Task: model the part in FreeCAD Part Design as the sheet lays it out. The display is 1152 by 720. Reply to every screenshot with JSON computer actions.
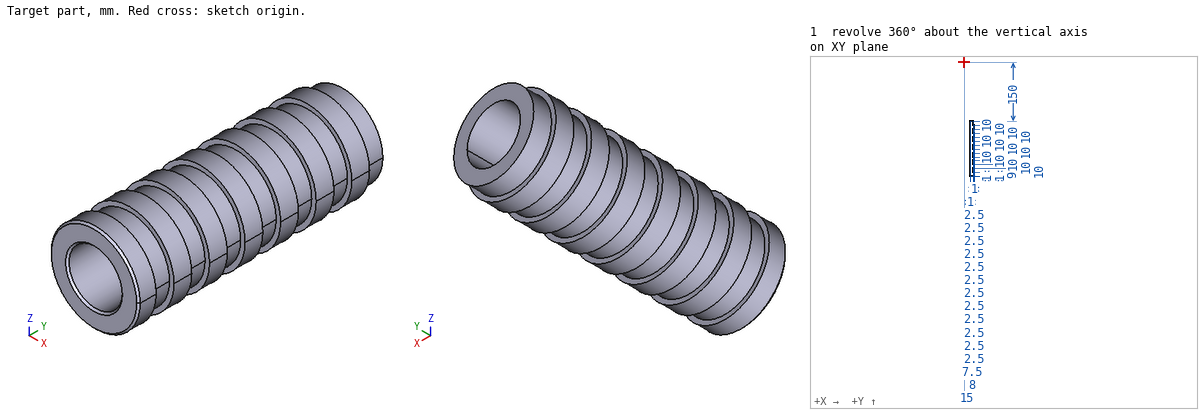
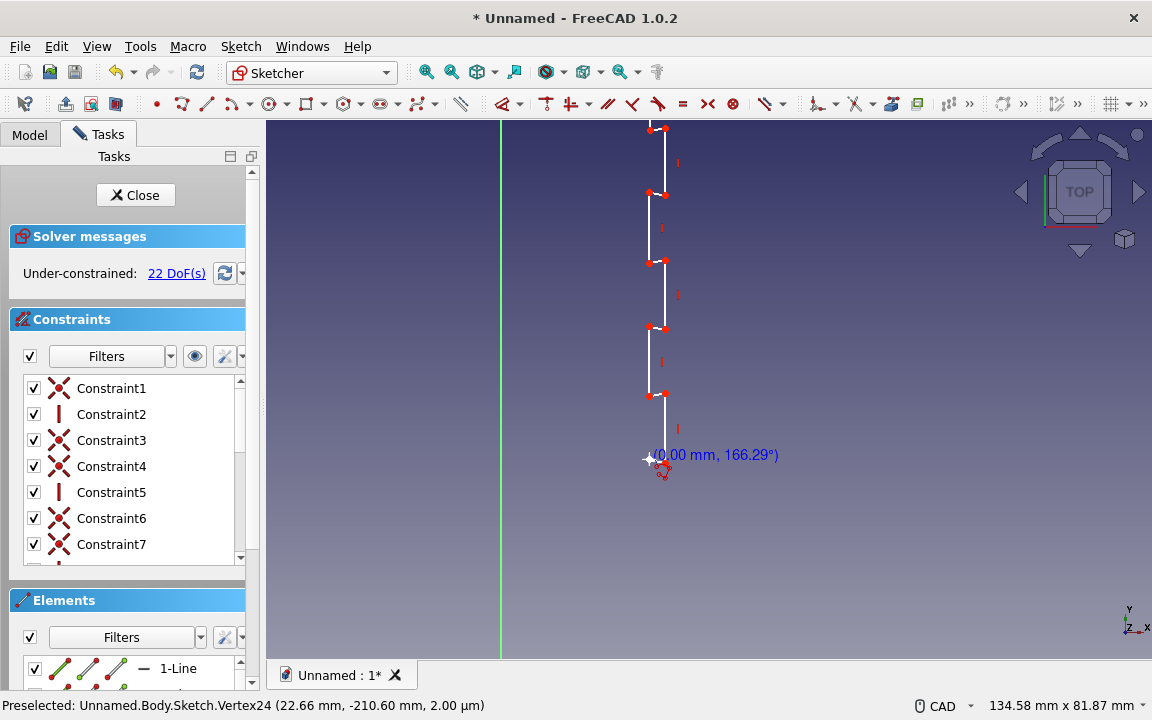
{"action": "scroll", "coordinate": [652, 461], "scroll_direction": "down", "scroll_amount": 9}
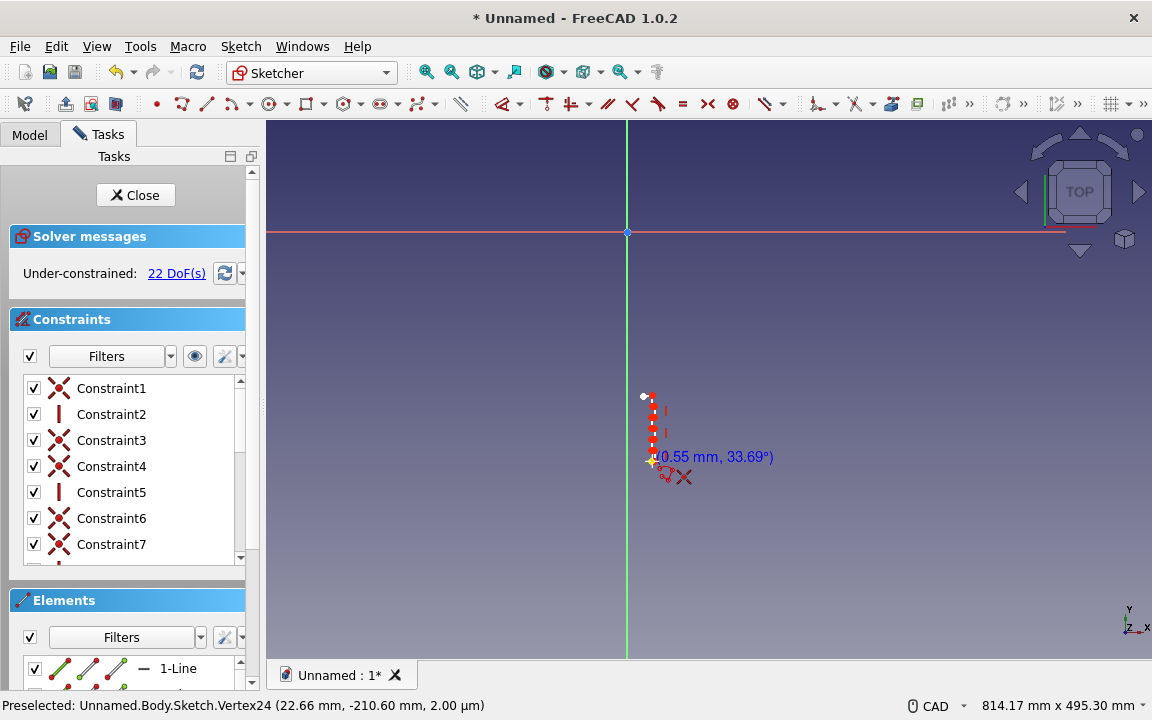
{"action": "scroll", "coordinate": [652, 472], "scroll_direction": "up", "scroll_amount": 2}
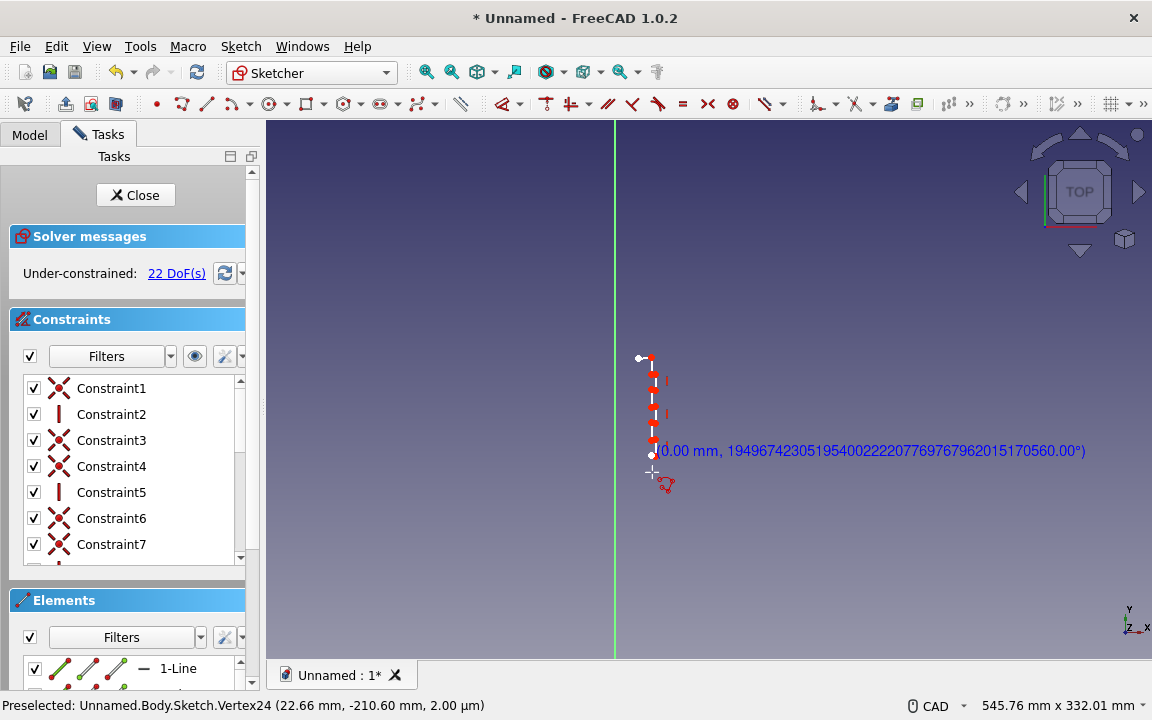
{"action": "left_click", "coordinate": [652, 471]}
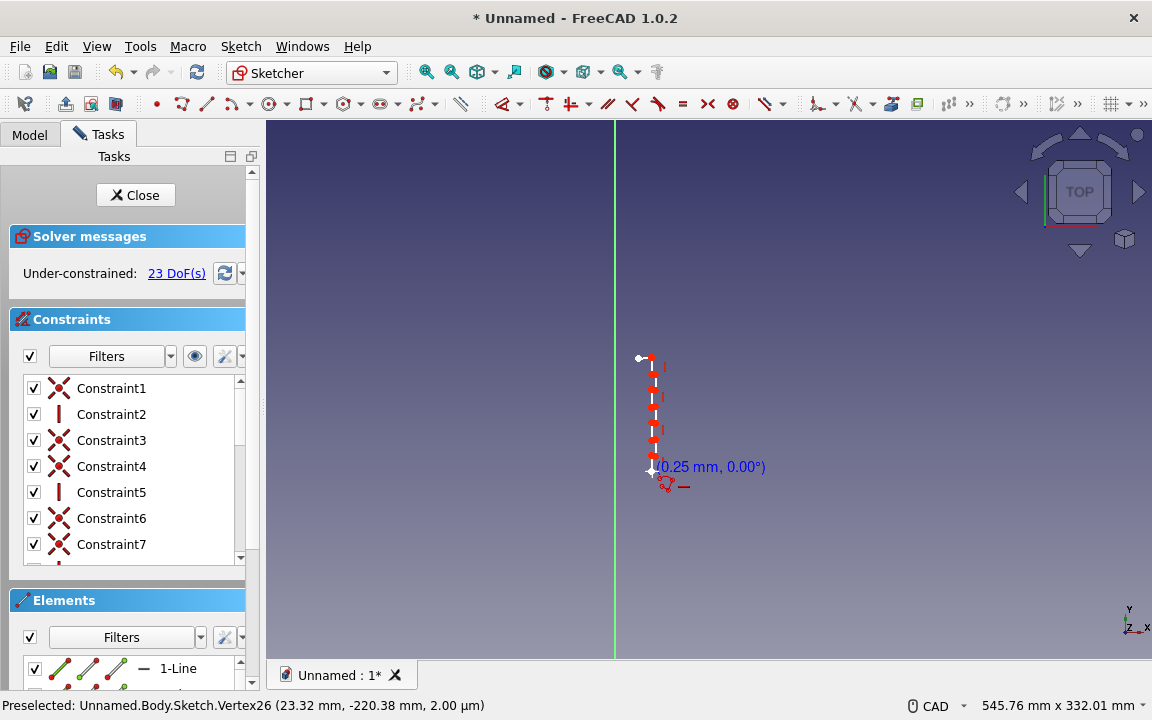
{"action": "scroll", "coordinate": [656, 471], "scroll_direction": "up", "scroll_amount": 7}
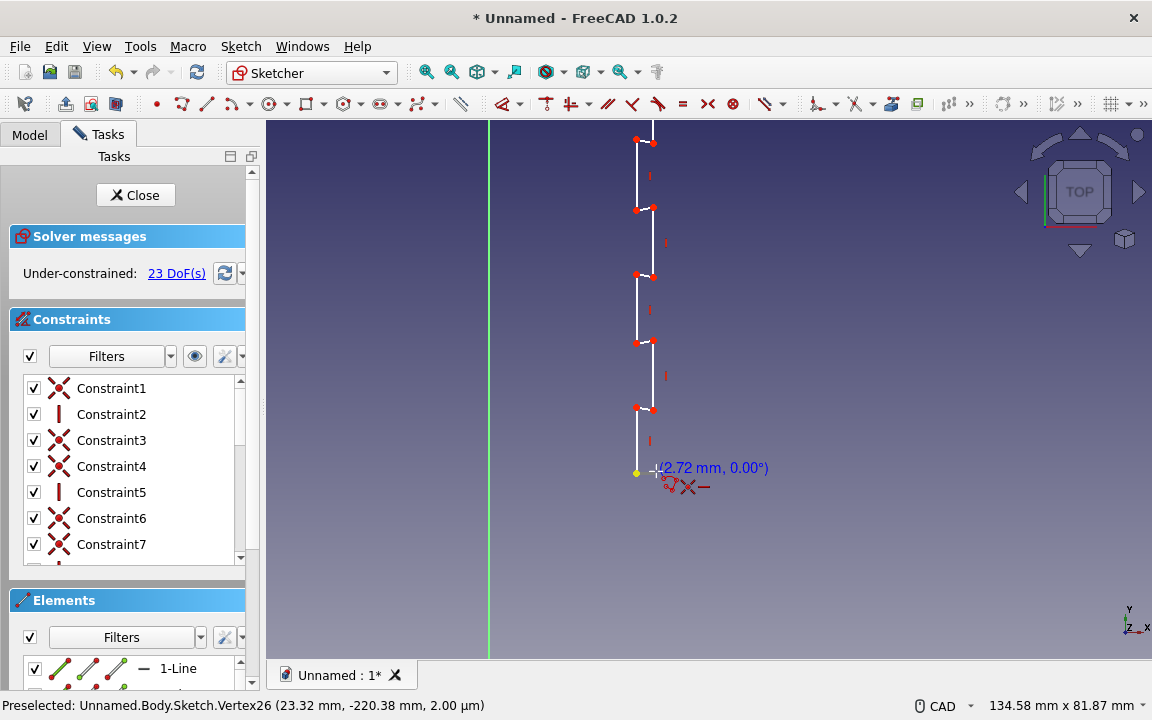
{"action": "left_click", "coordinate": [653, 469]}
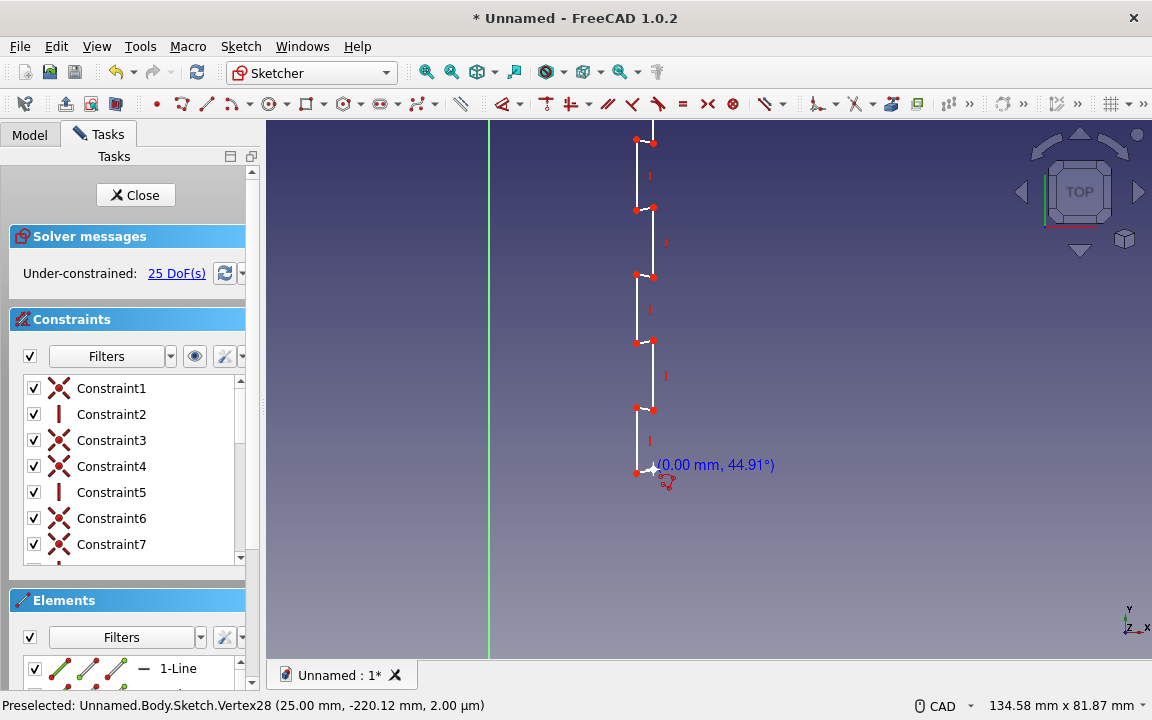
{"action": "scroll", "coordinate": [654, 471], "scroll_direction": "down", "scroll_amount": 9}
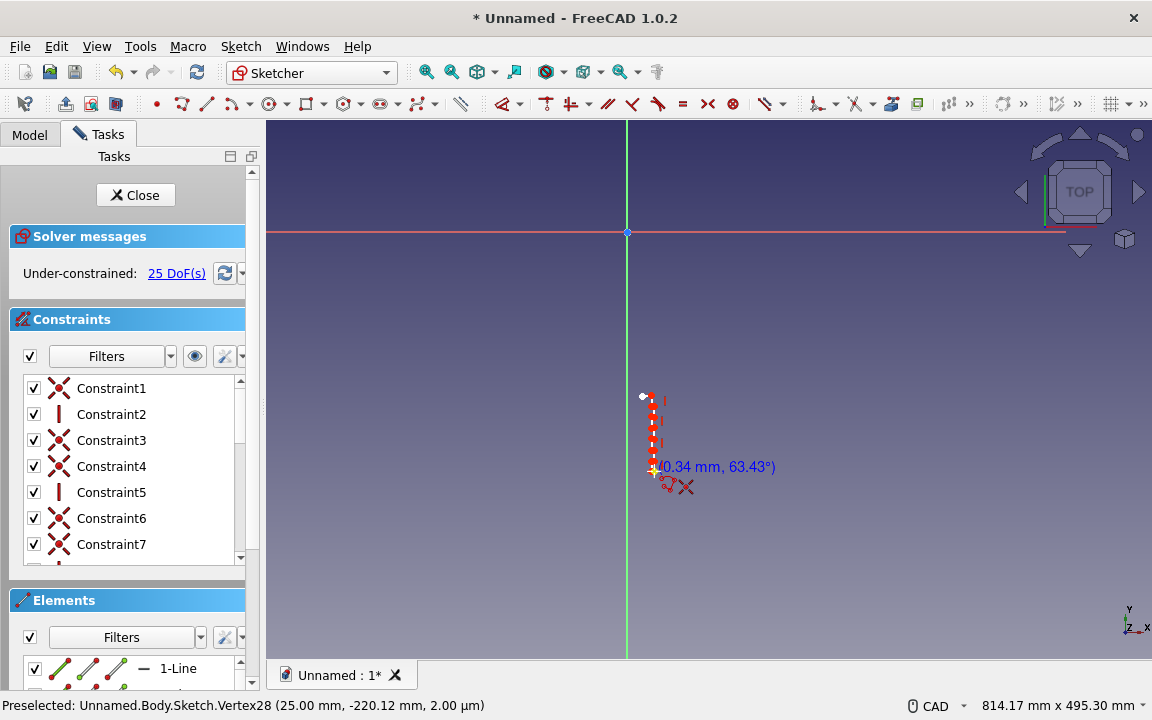
{"action": "scroll", "coordinate": [654, 482], "scroll_direction": "up", "scroll_amount": 2}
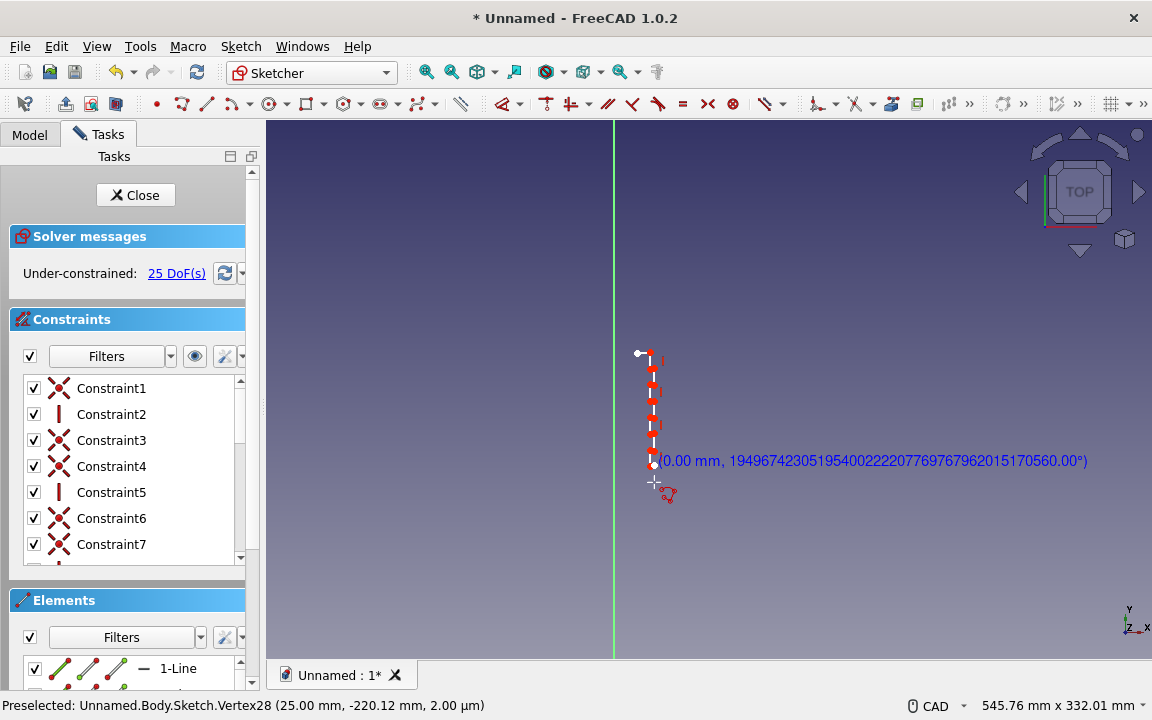
{"action": "left_click", "coordinate": [654, 482]}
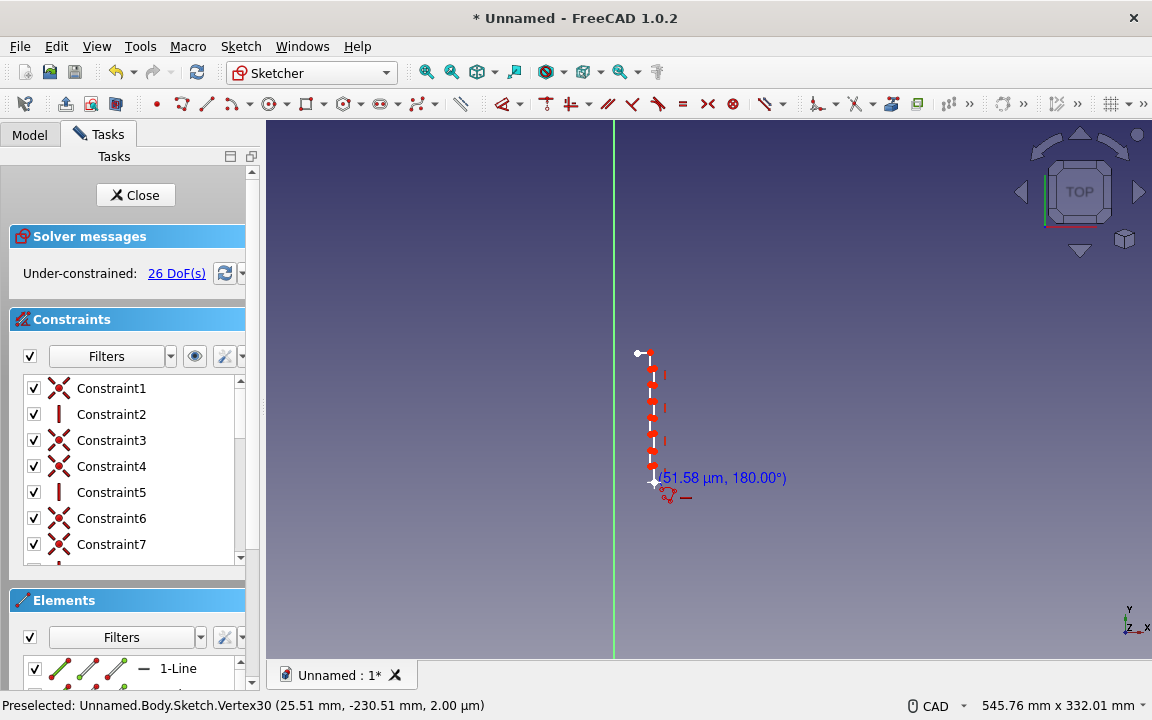
{"action": "scroll", "coordinate": [650, 482], "scroll_direction": "up", "scroll_amount": 7}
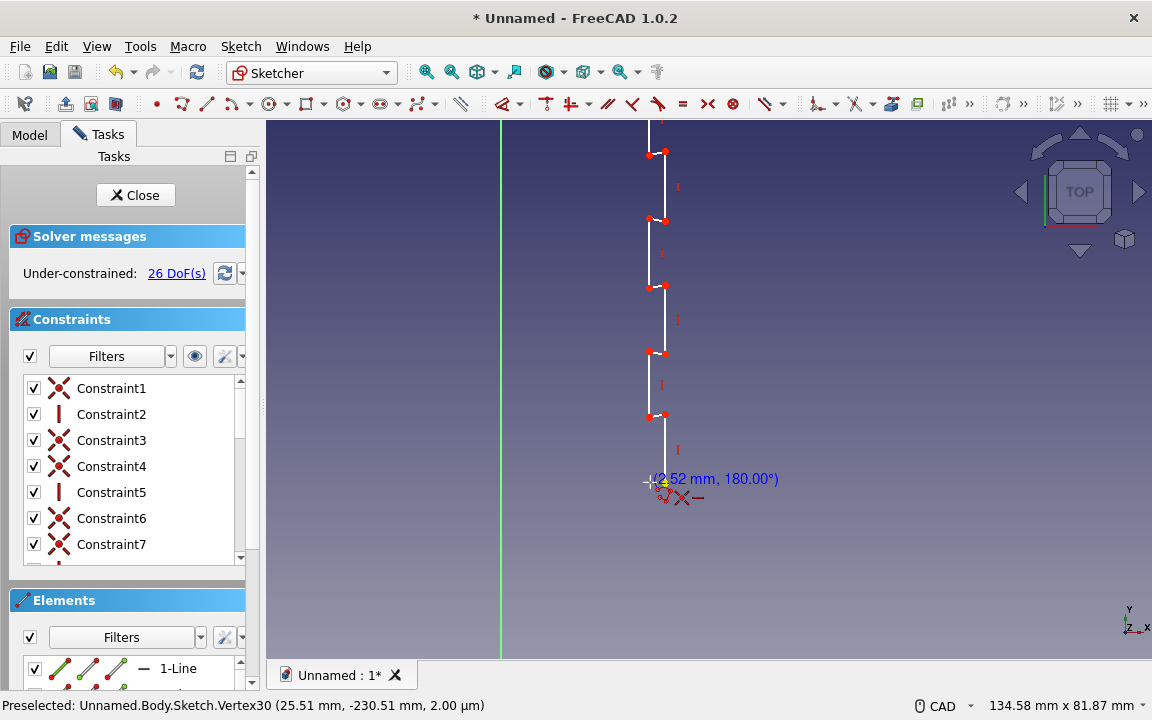
{"action": "left_click", "coordinate": [649, 480]}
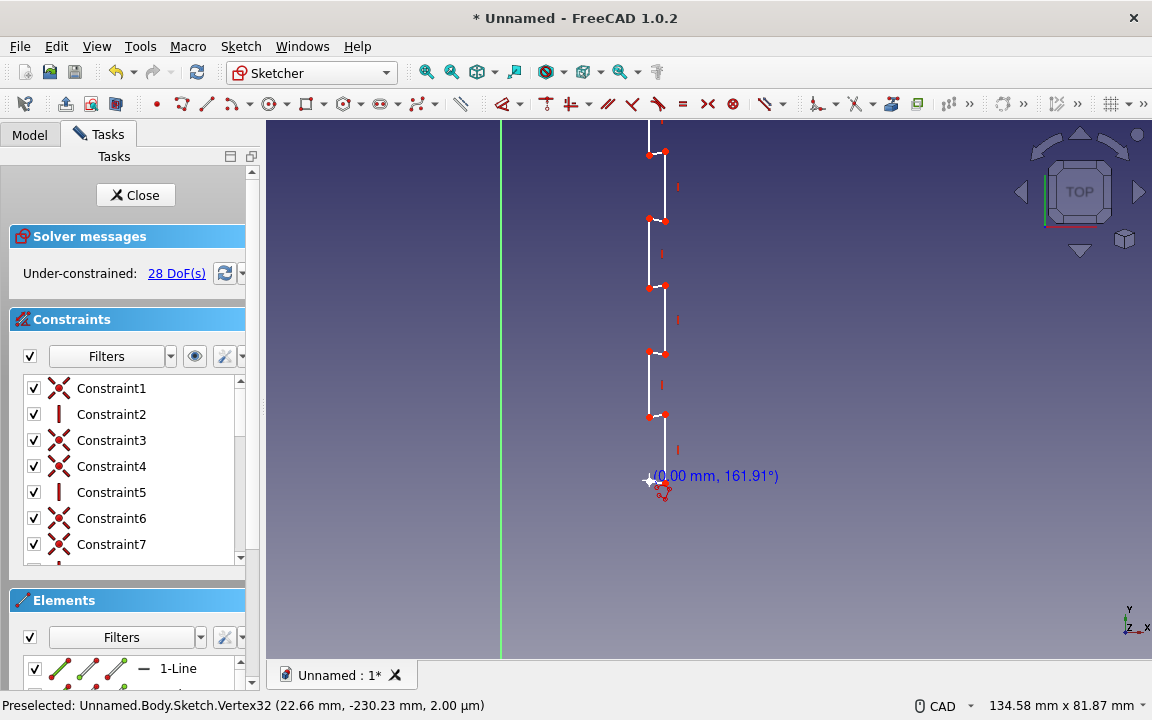
{"action": "scroll", "coordinate": [652, 482], "scroll_direction": "down", "scroll_amount": 9}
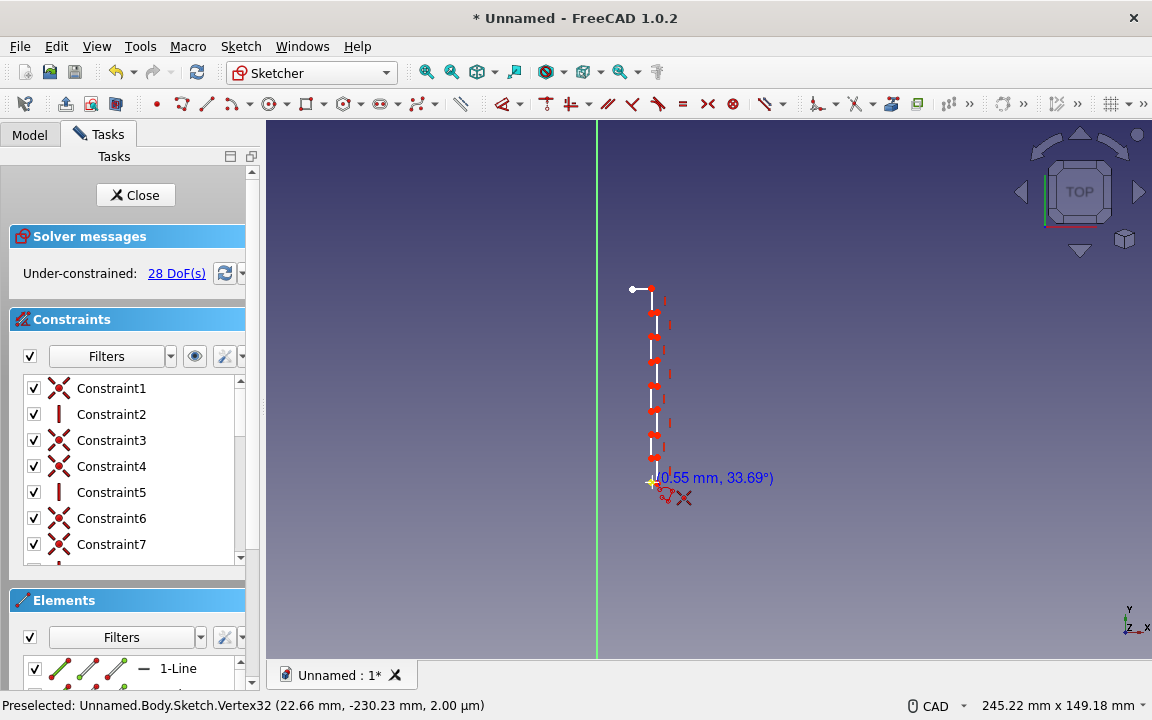
{"action": "scroll", "coordinate": [652, 493], "scroll_direction": "up", "scroll_amount": 2}